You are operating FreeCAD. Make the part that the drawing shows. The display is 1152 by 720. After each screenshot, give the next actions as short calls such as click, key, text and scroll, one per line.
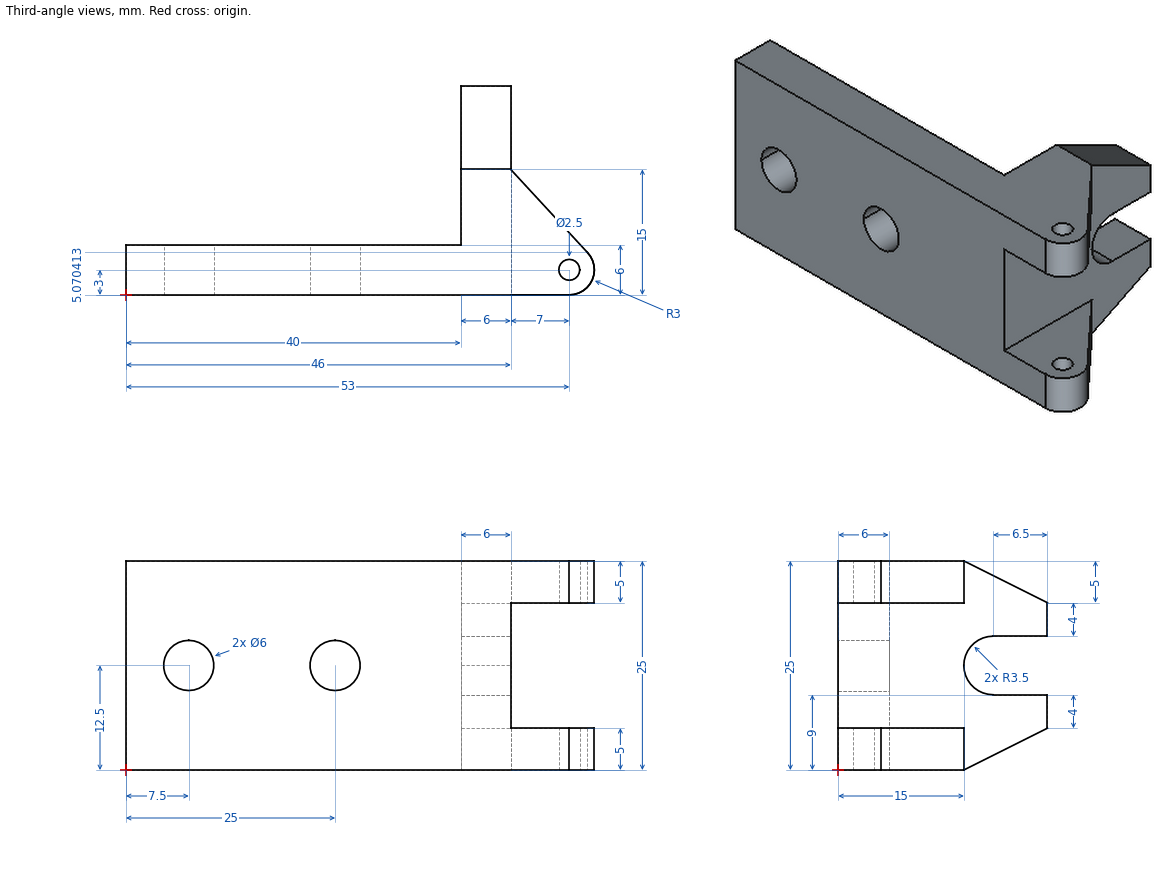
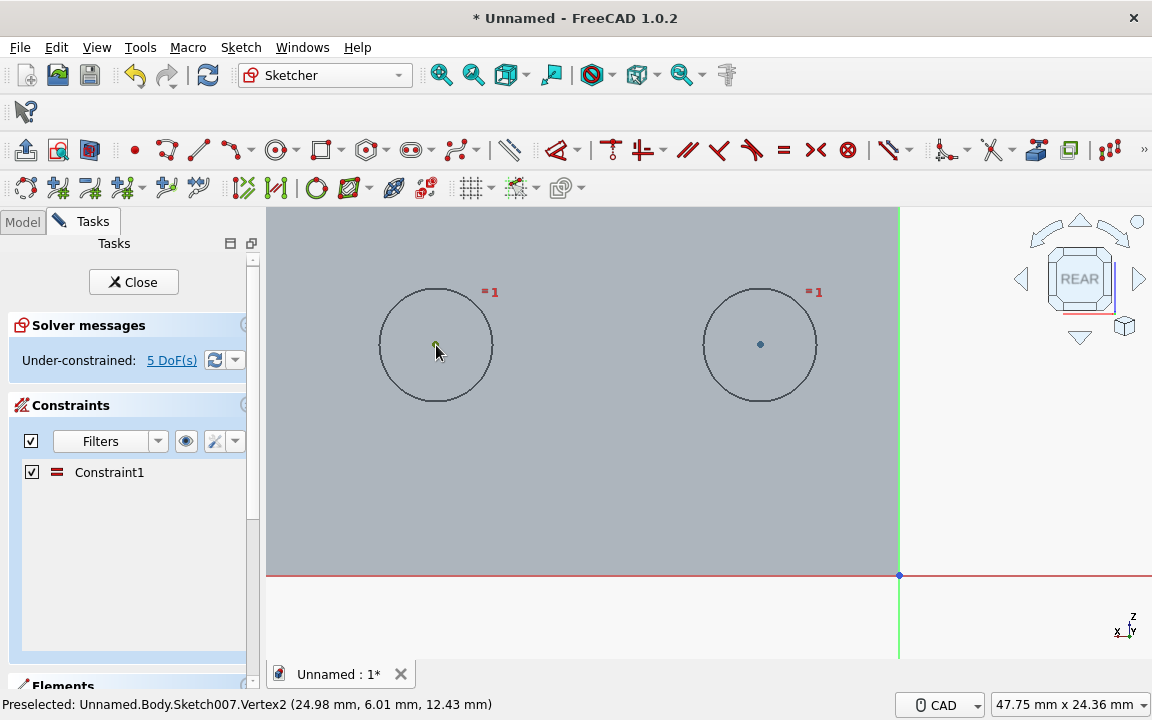
click(666, 150)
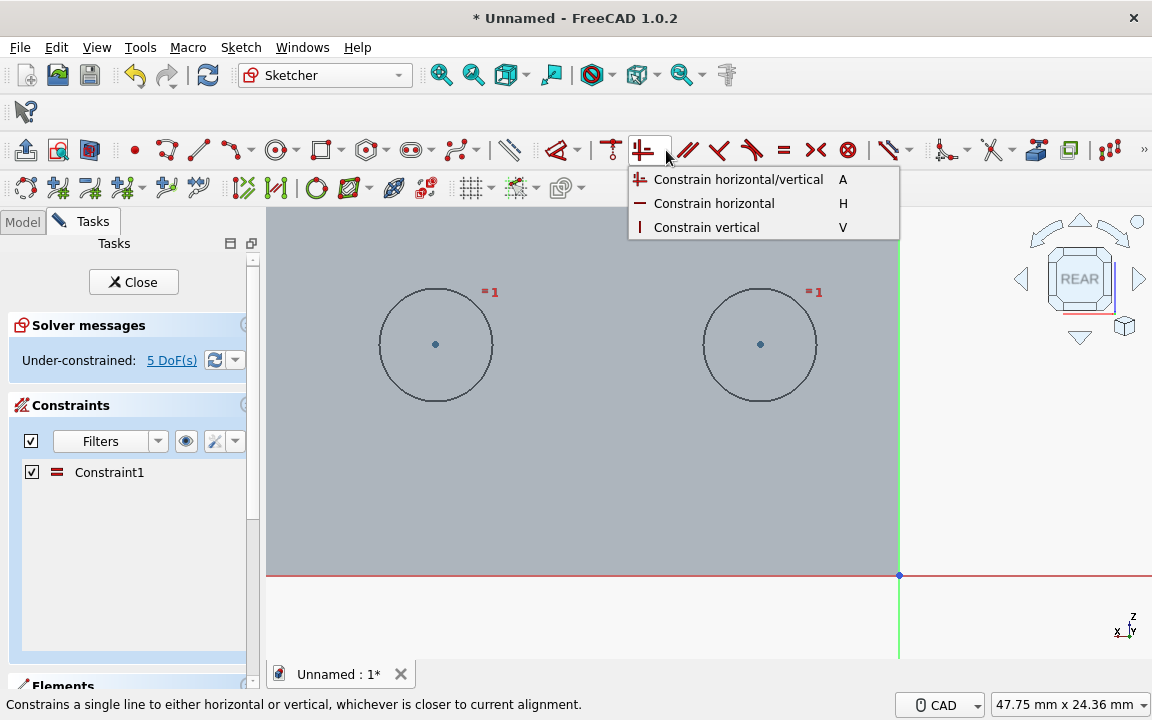
click(764, 203)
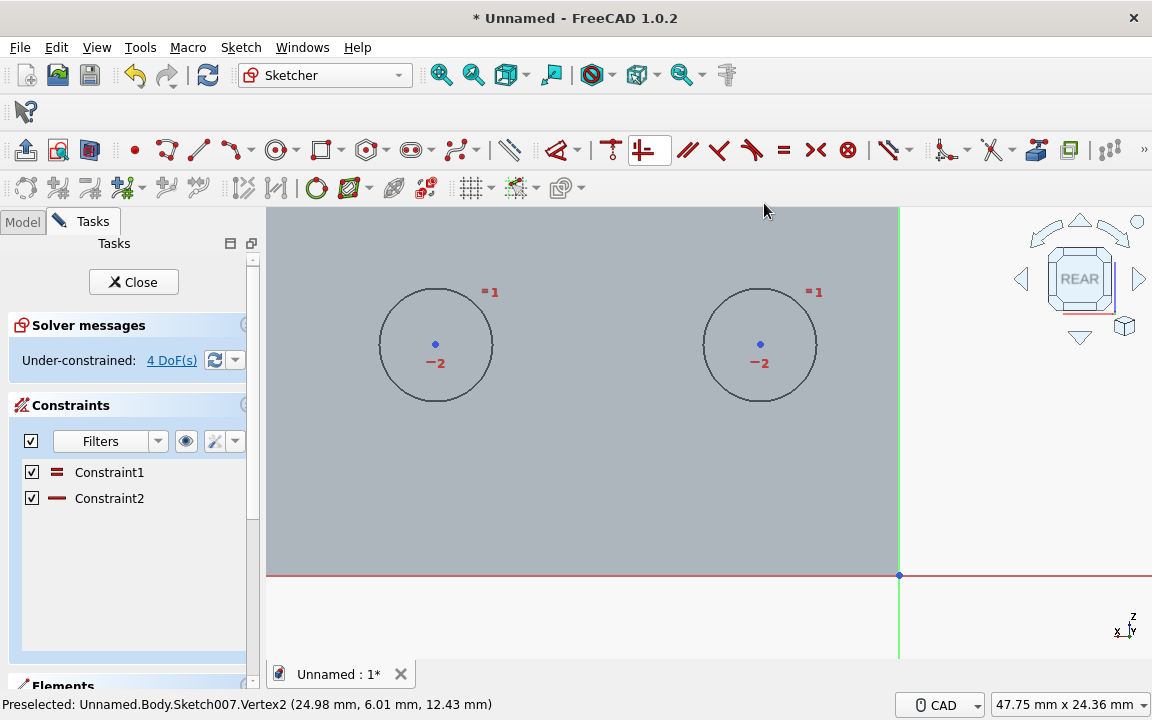
key(d)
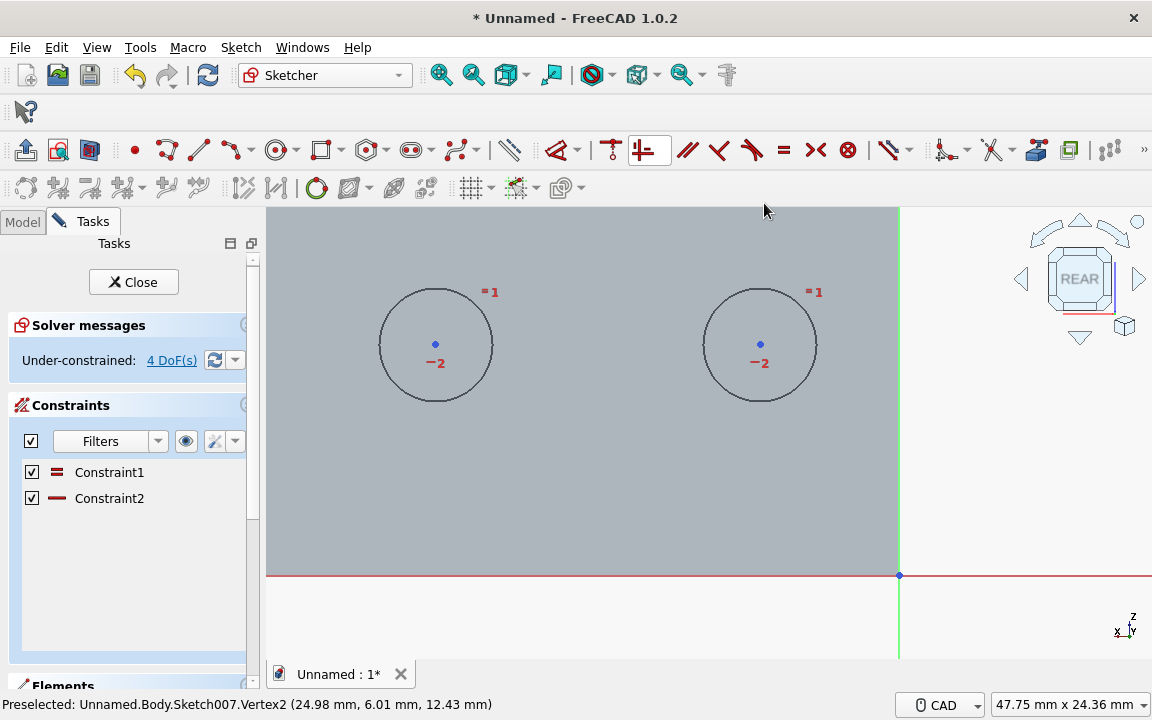
click(800, 305)
click(823, 282)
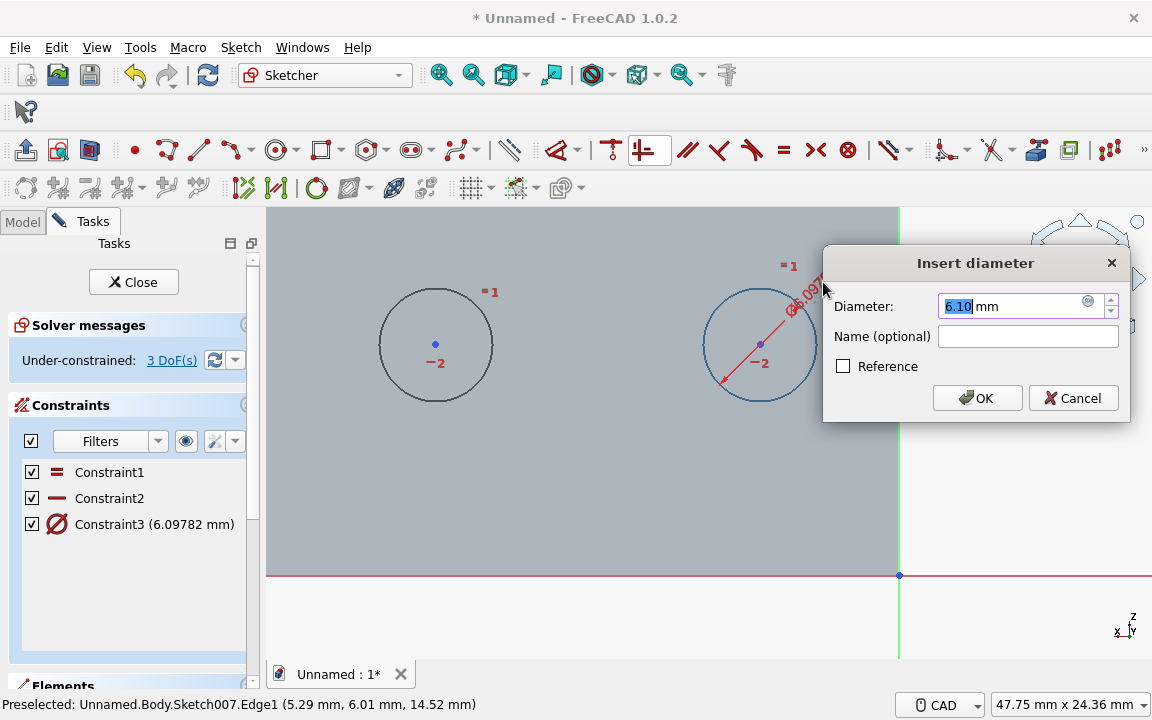
text(6)
key(Return)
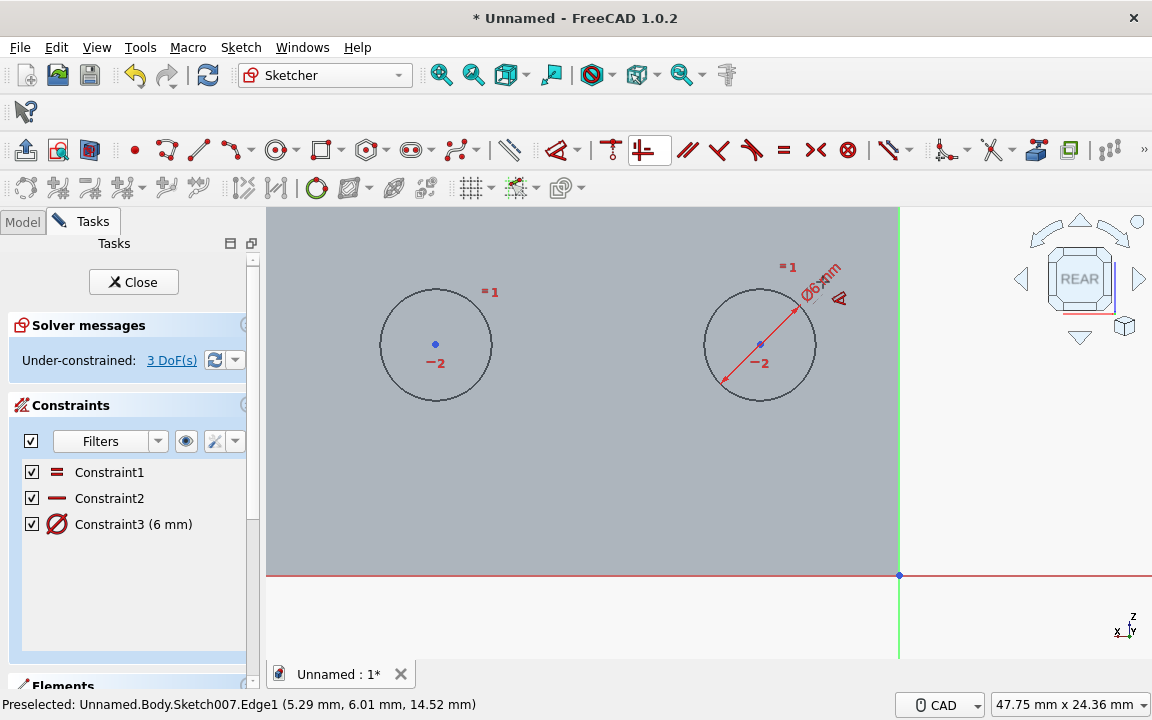
click(436, 345)
click(668, 610)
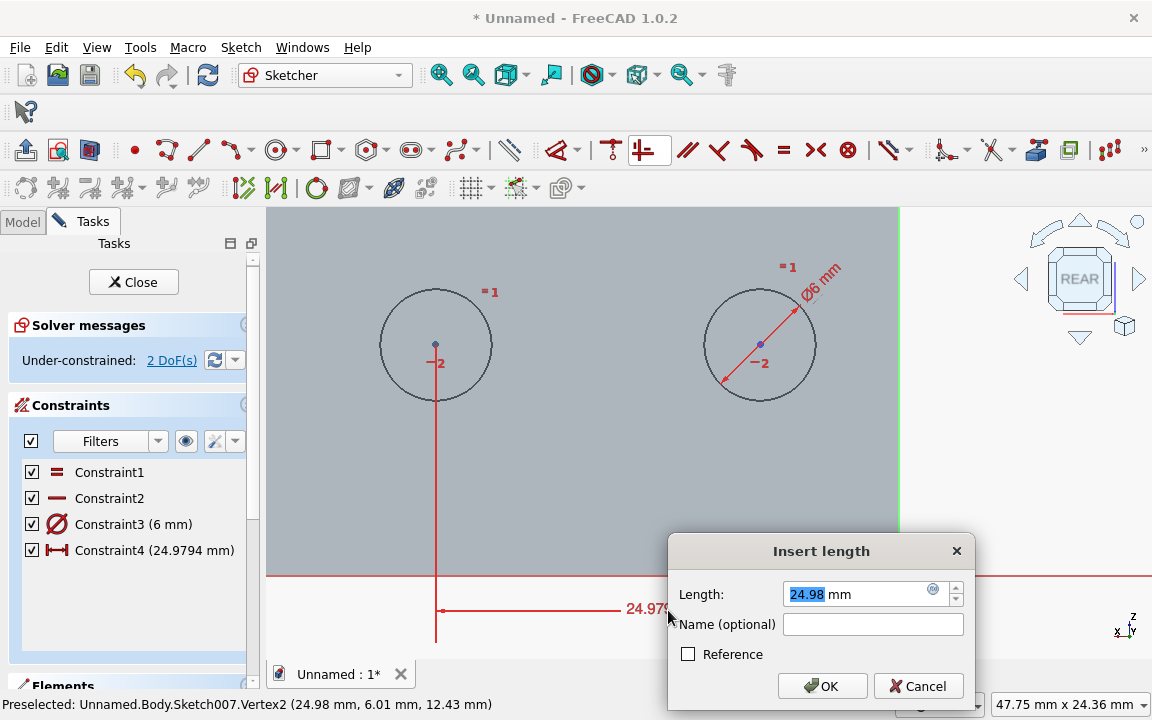
text(25)
key(Return)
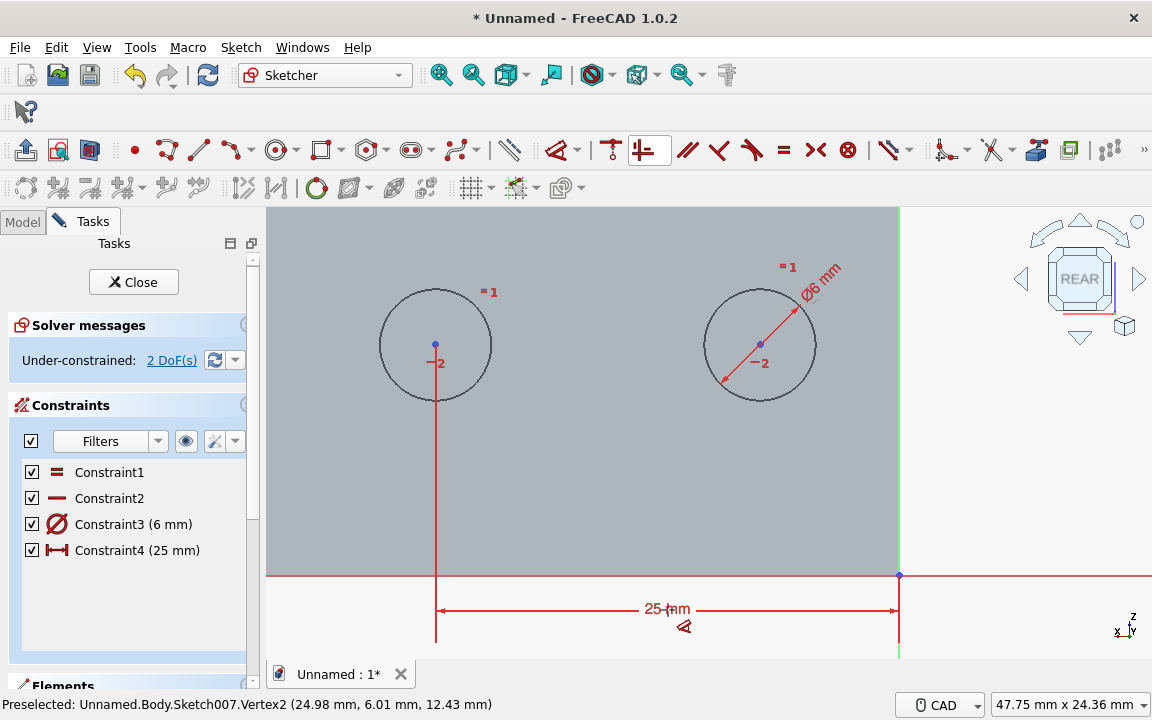
click(760, 345)
click(830, 610)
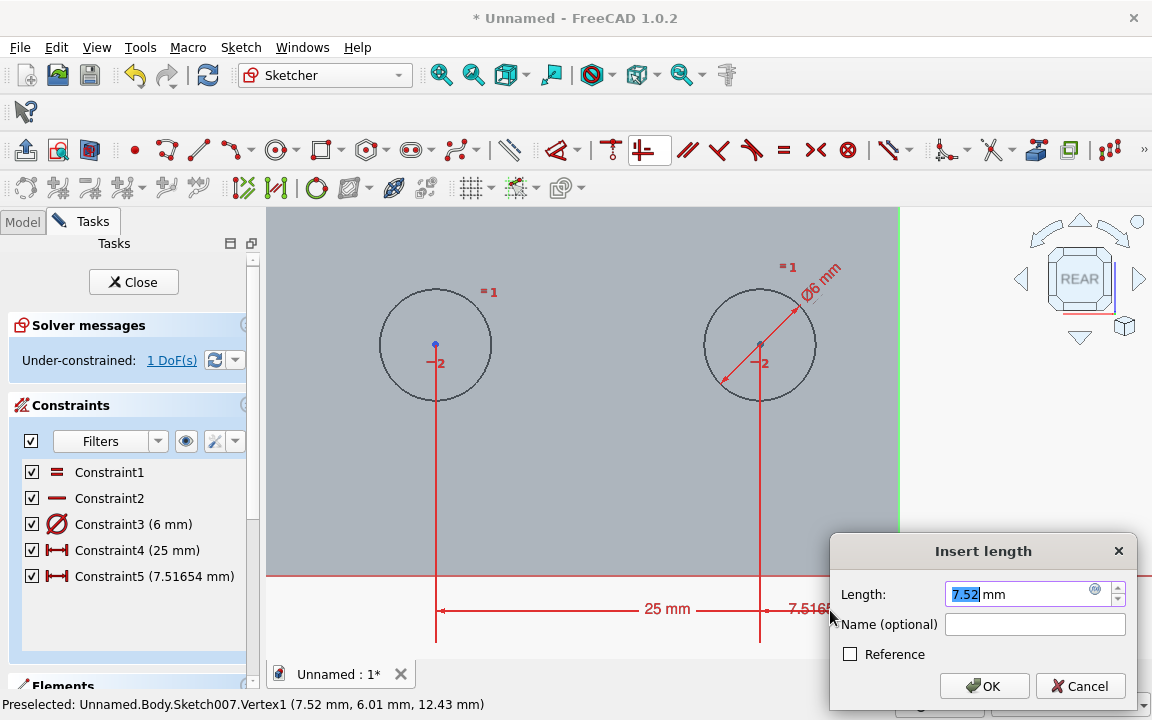
text(7.5)
key(Return)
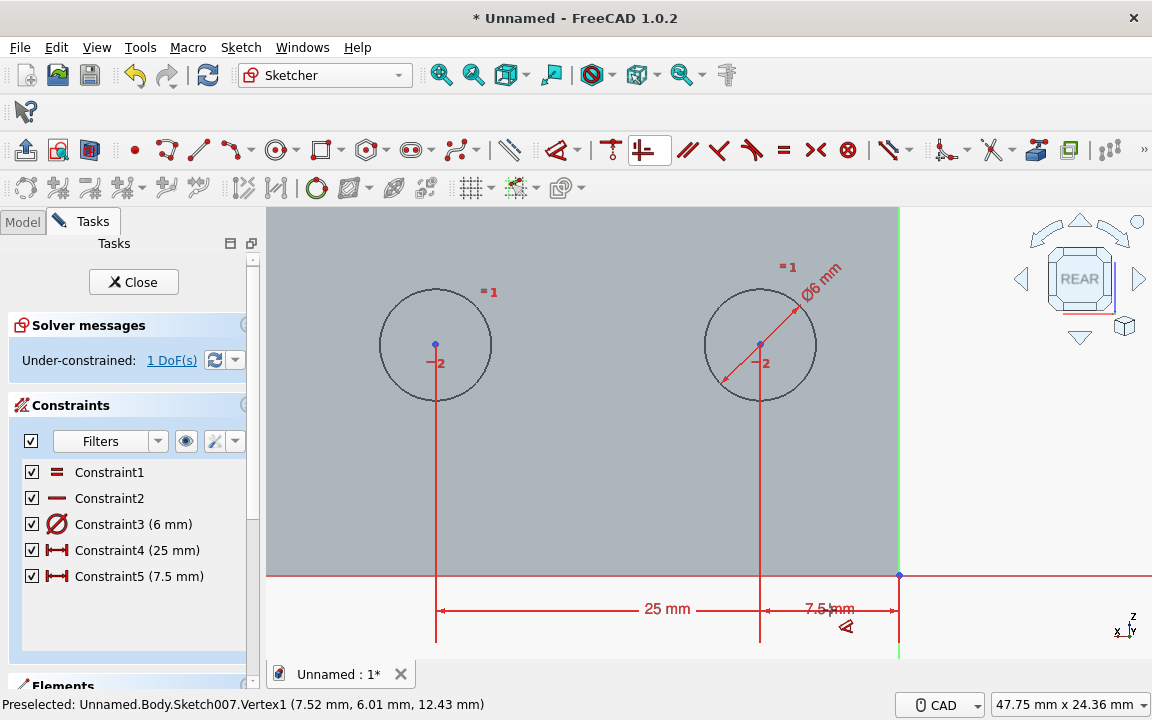
click(760, 345)
click(933, 460)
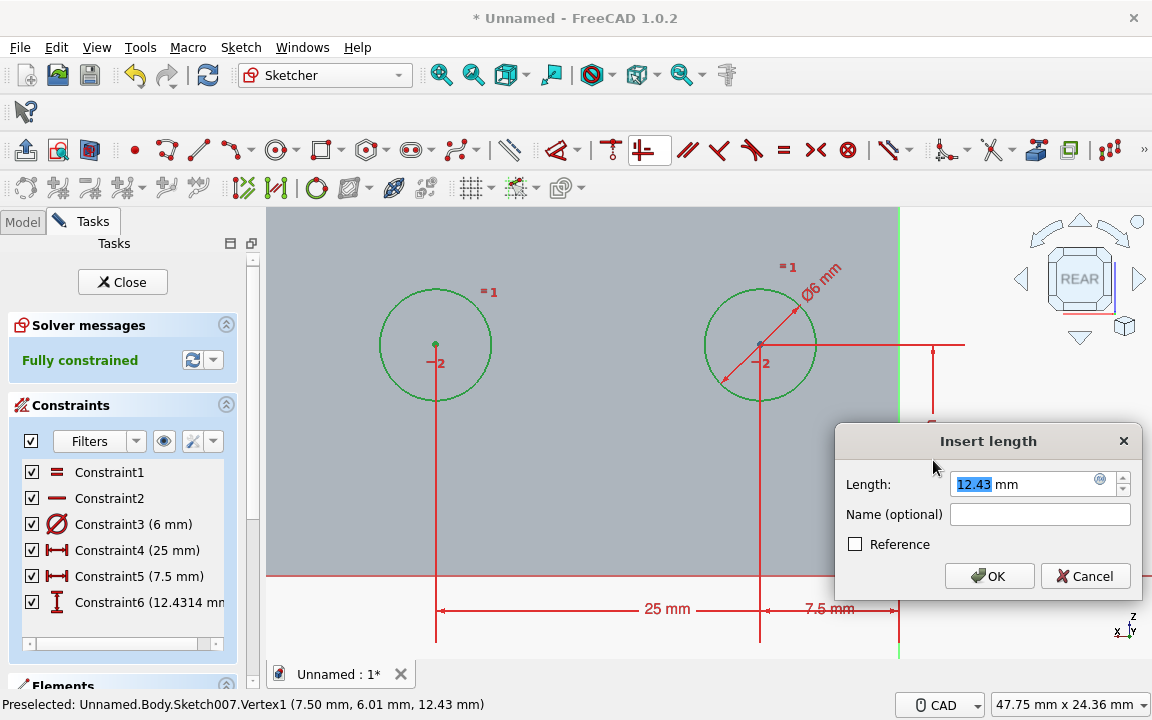
text(12.5)
key(Return)
key(Escape)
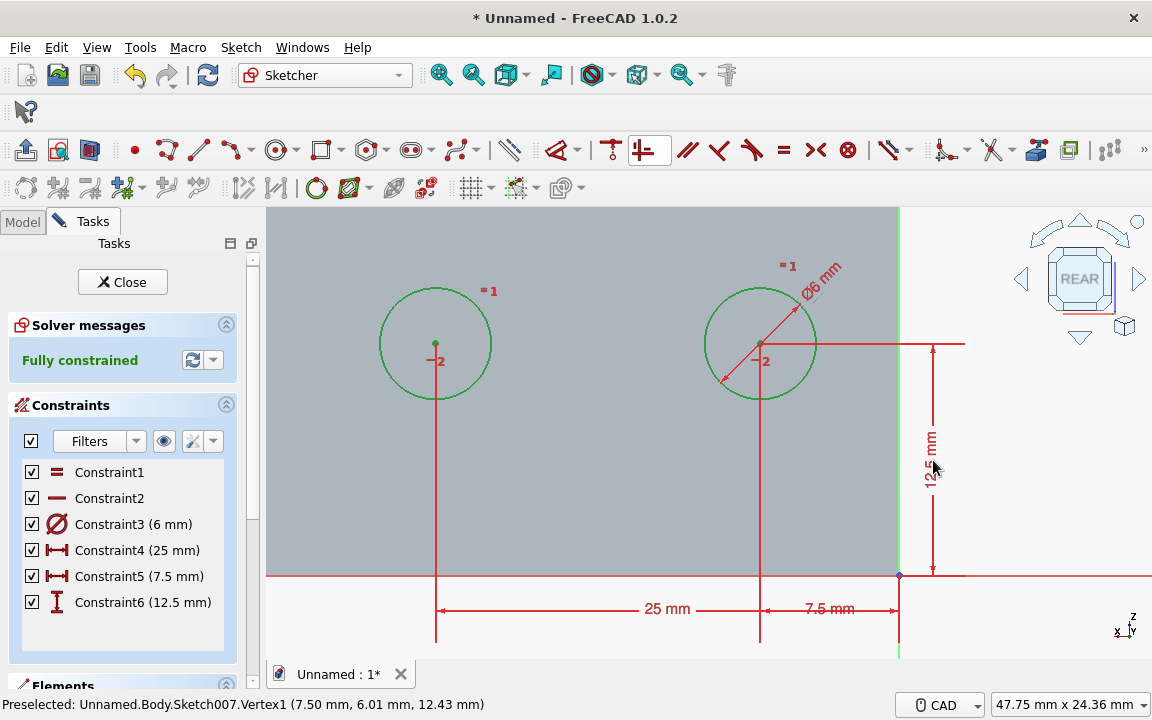
click(123, 282)